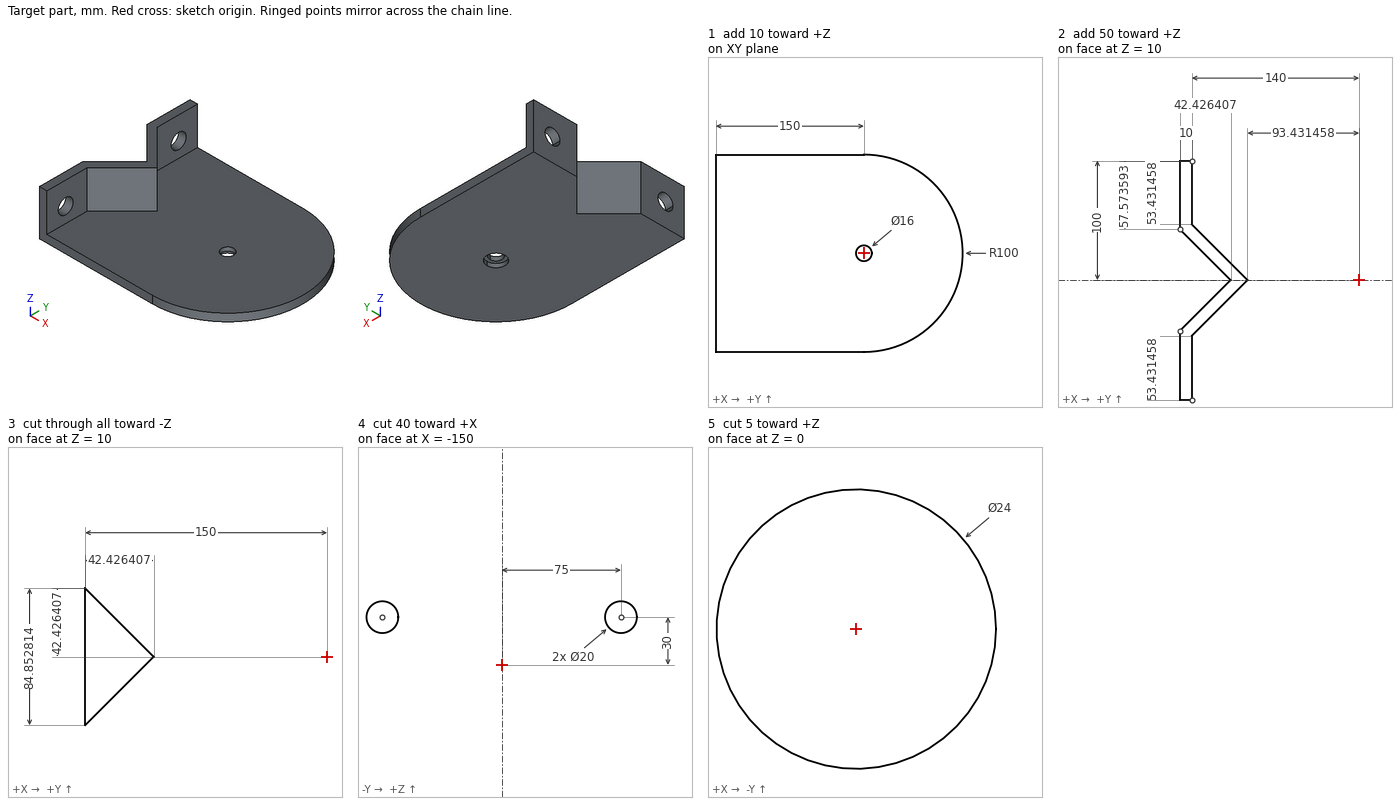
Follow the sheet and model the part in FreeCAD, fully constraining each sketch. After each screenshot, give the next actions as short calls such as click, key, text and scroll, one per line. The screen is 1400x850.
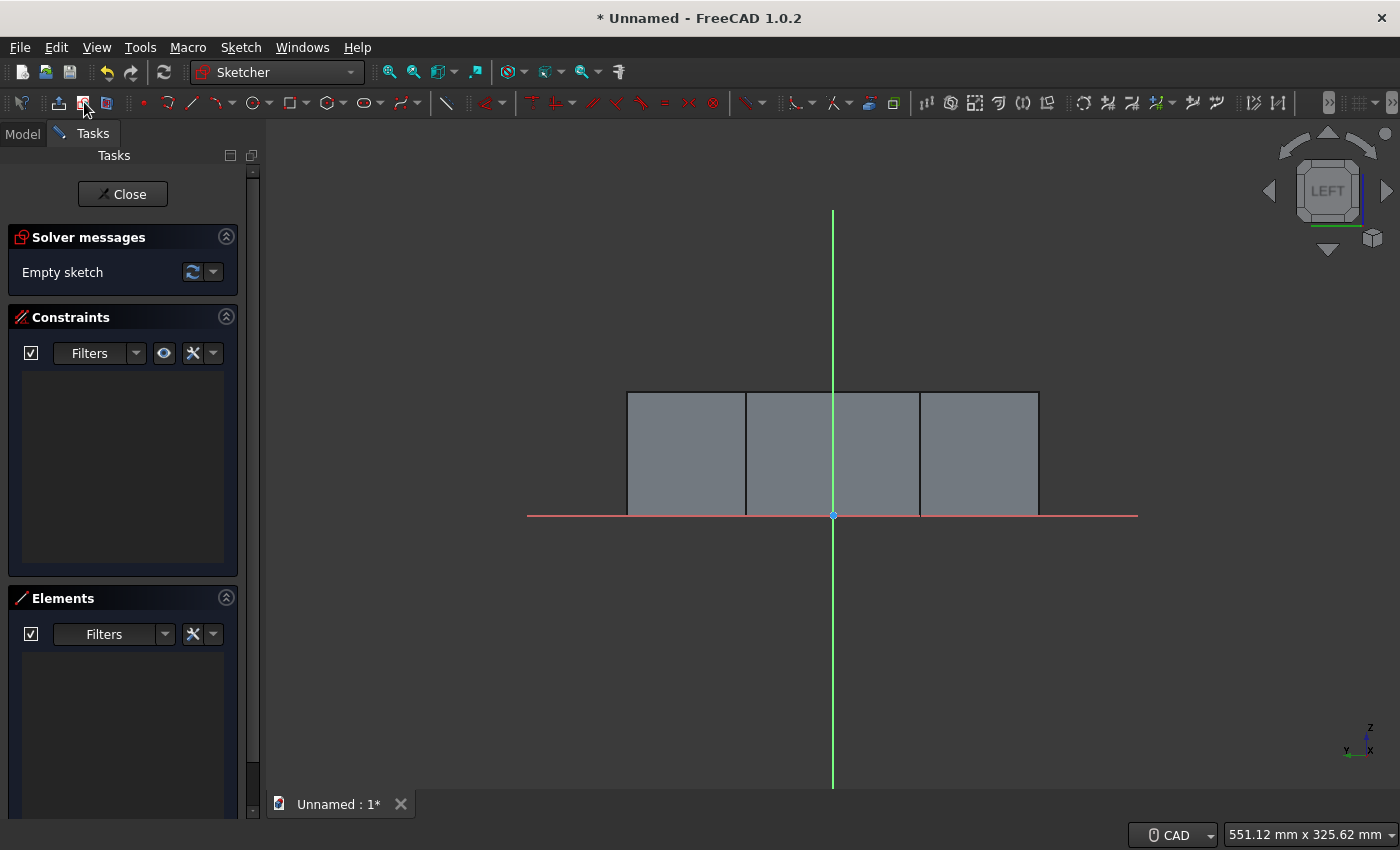
scroll(916, 500, up, 3)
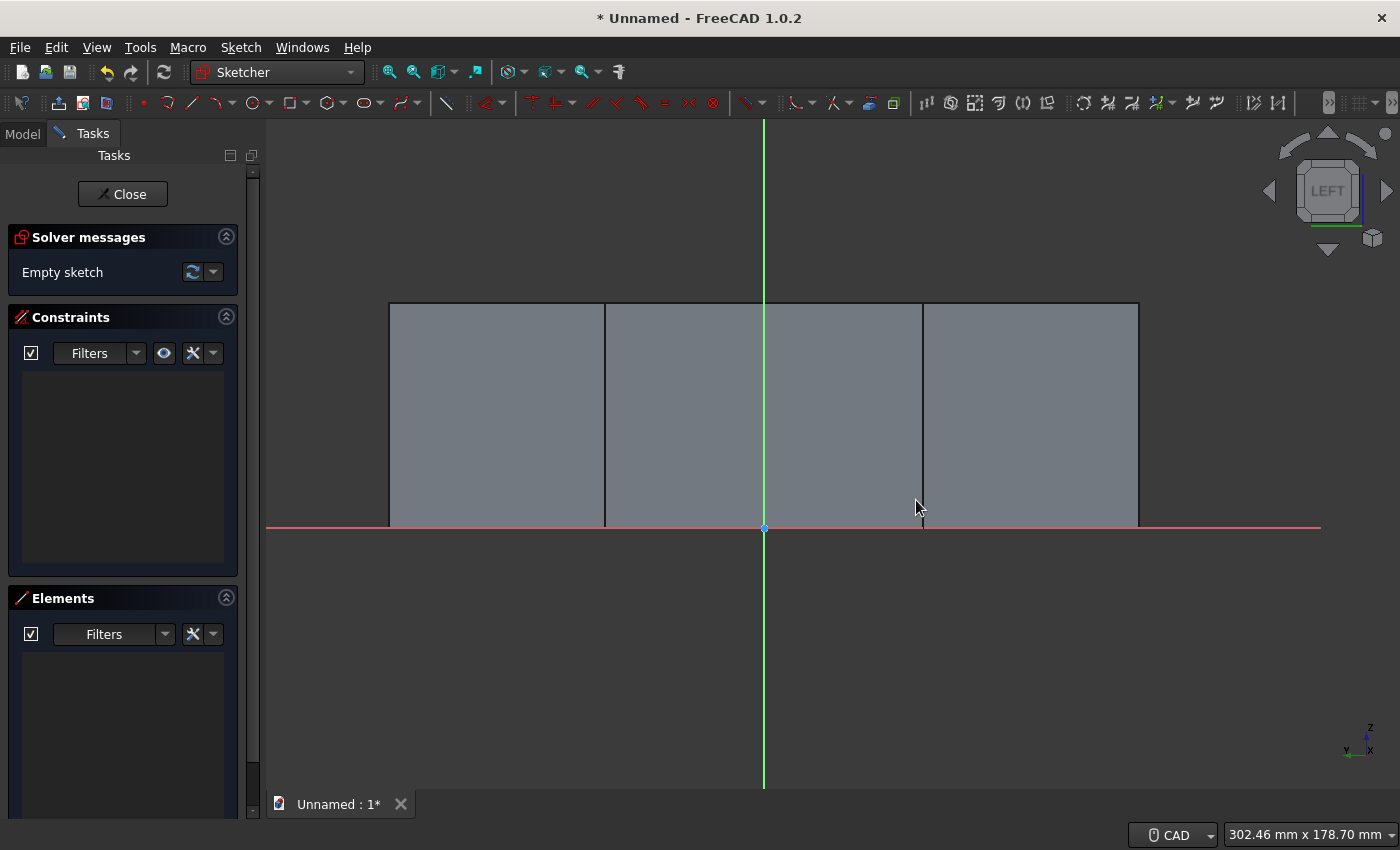
click(254, 104)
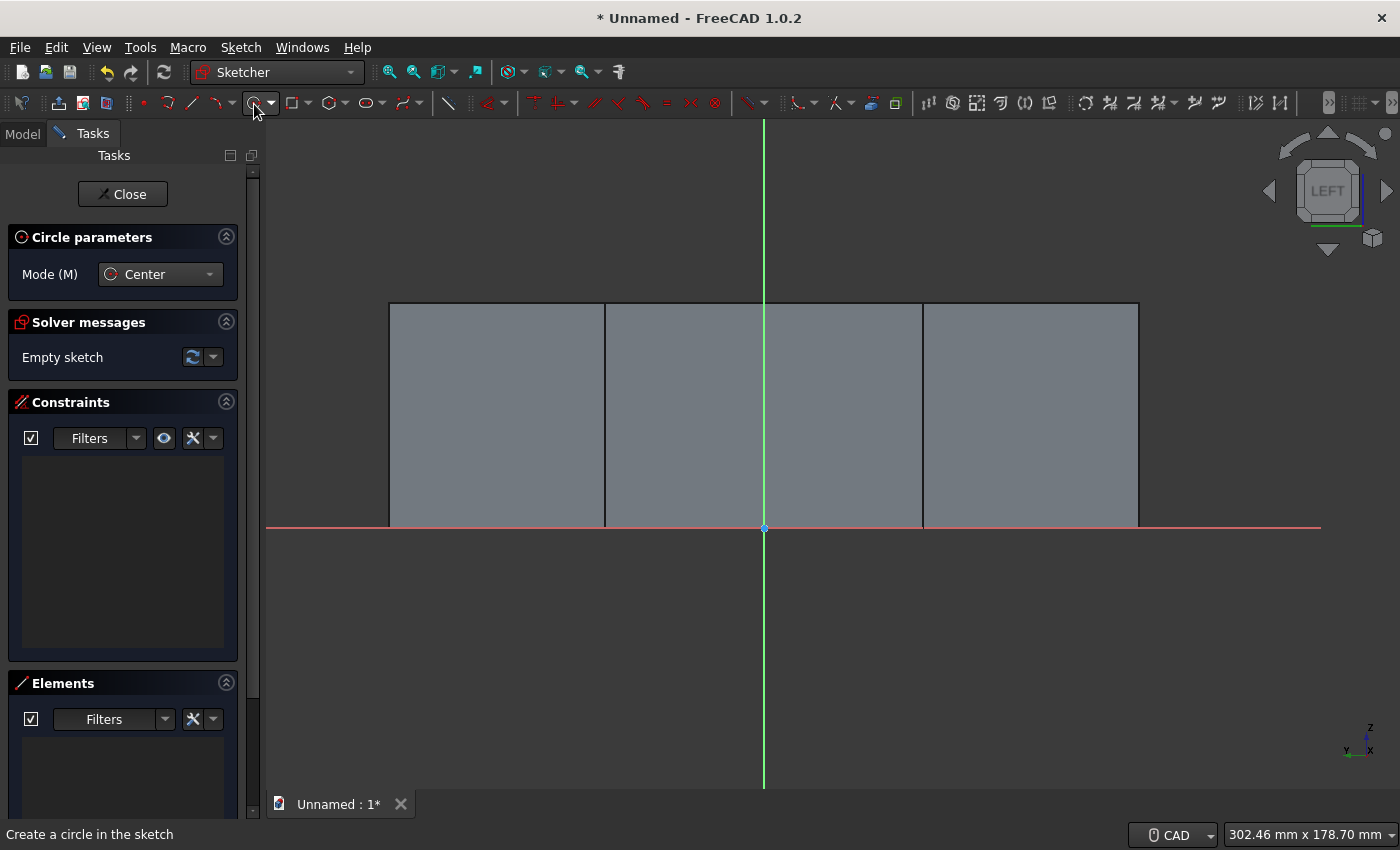
click(1045, 416)
click(1072, 389)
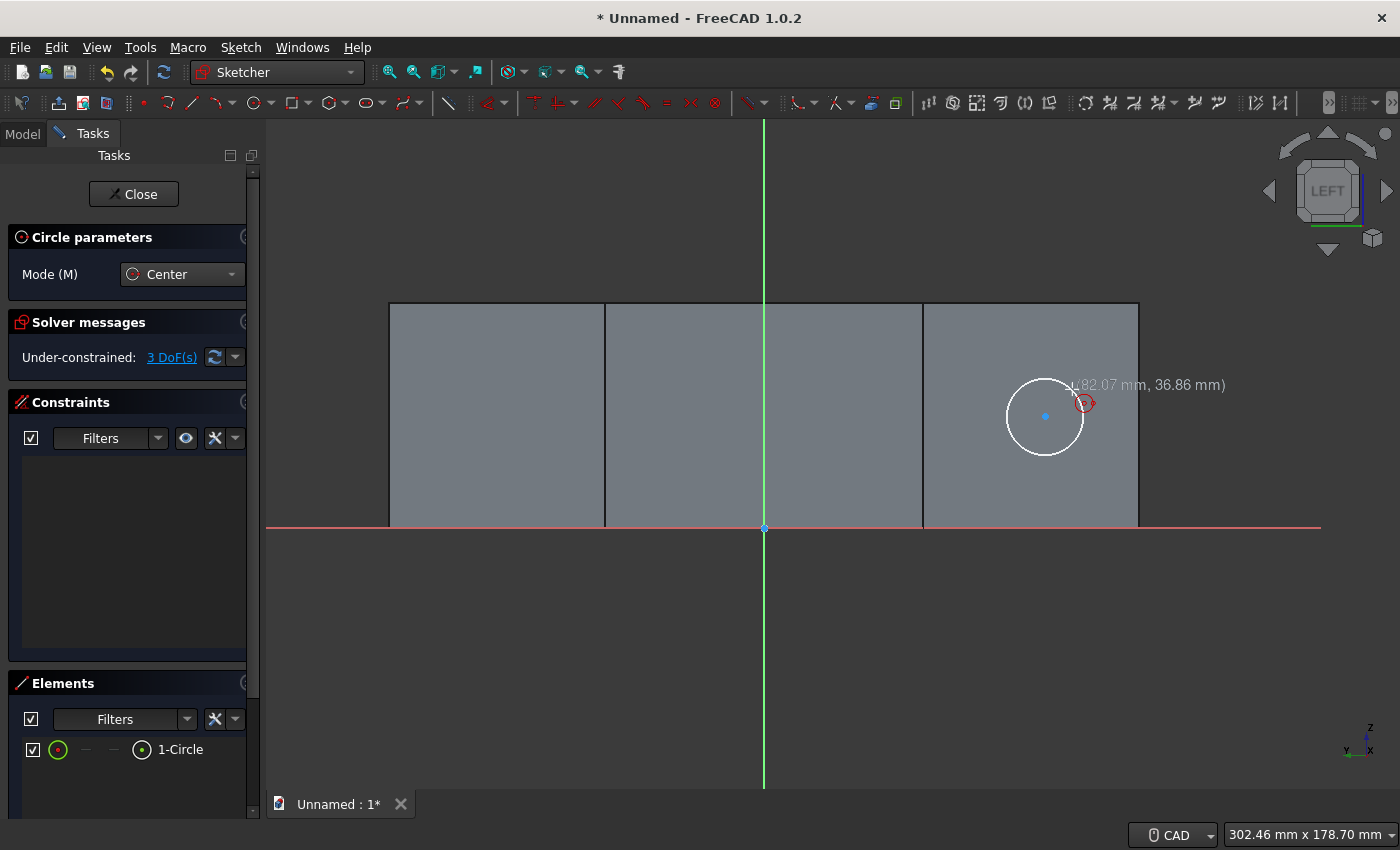
click(483, 416)
click(510, 389)
key(Escape)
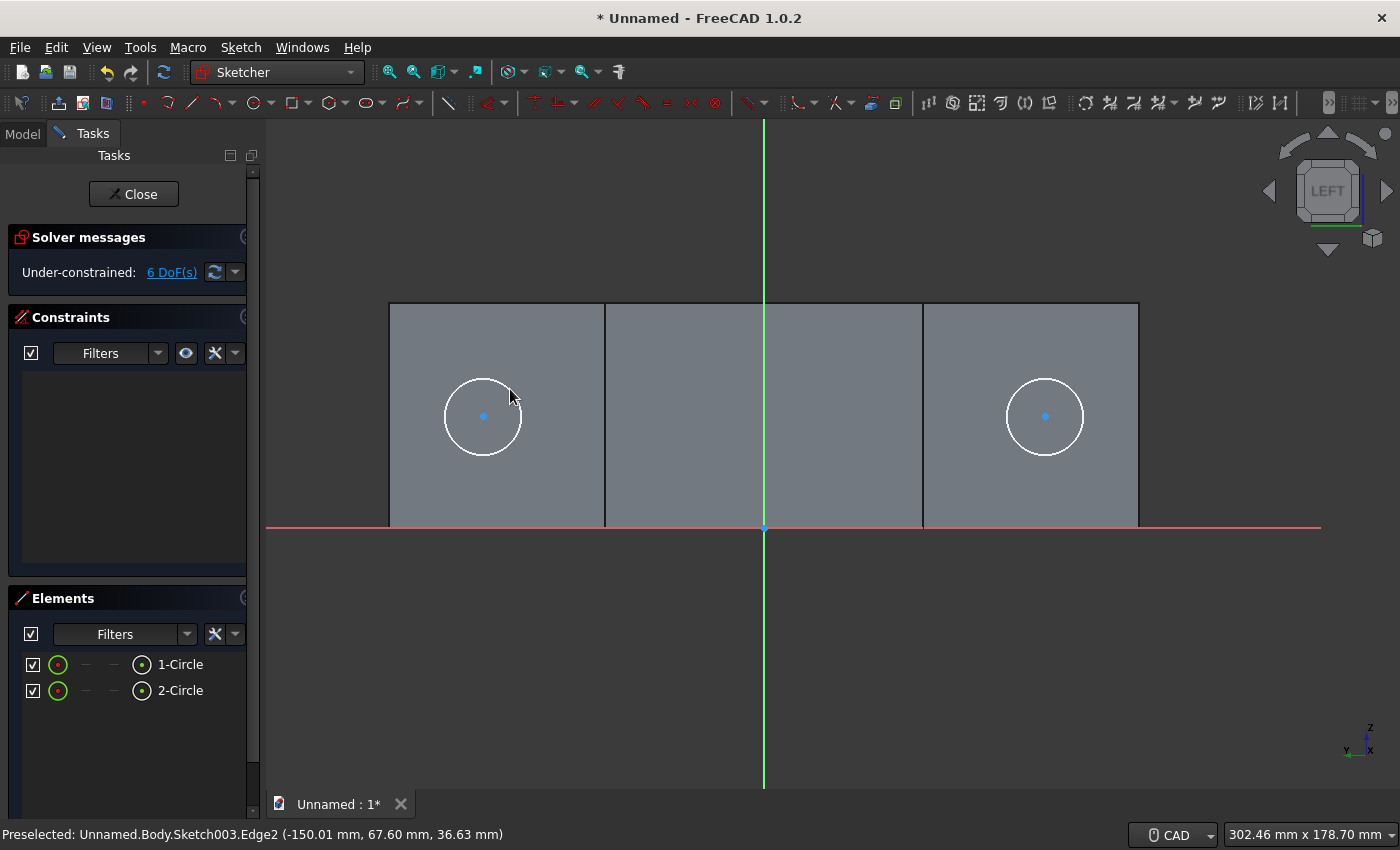
click(1072, 390)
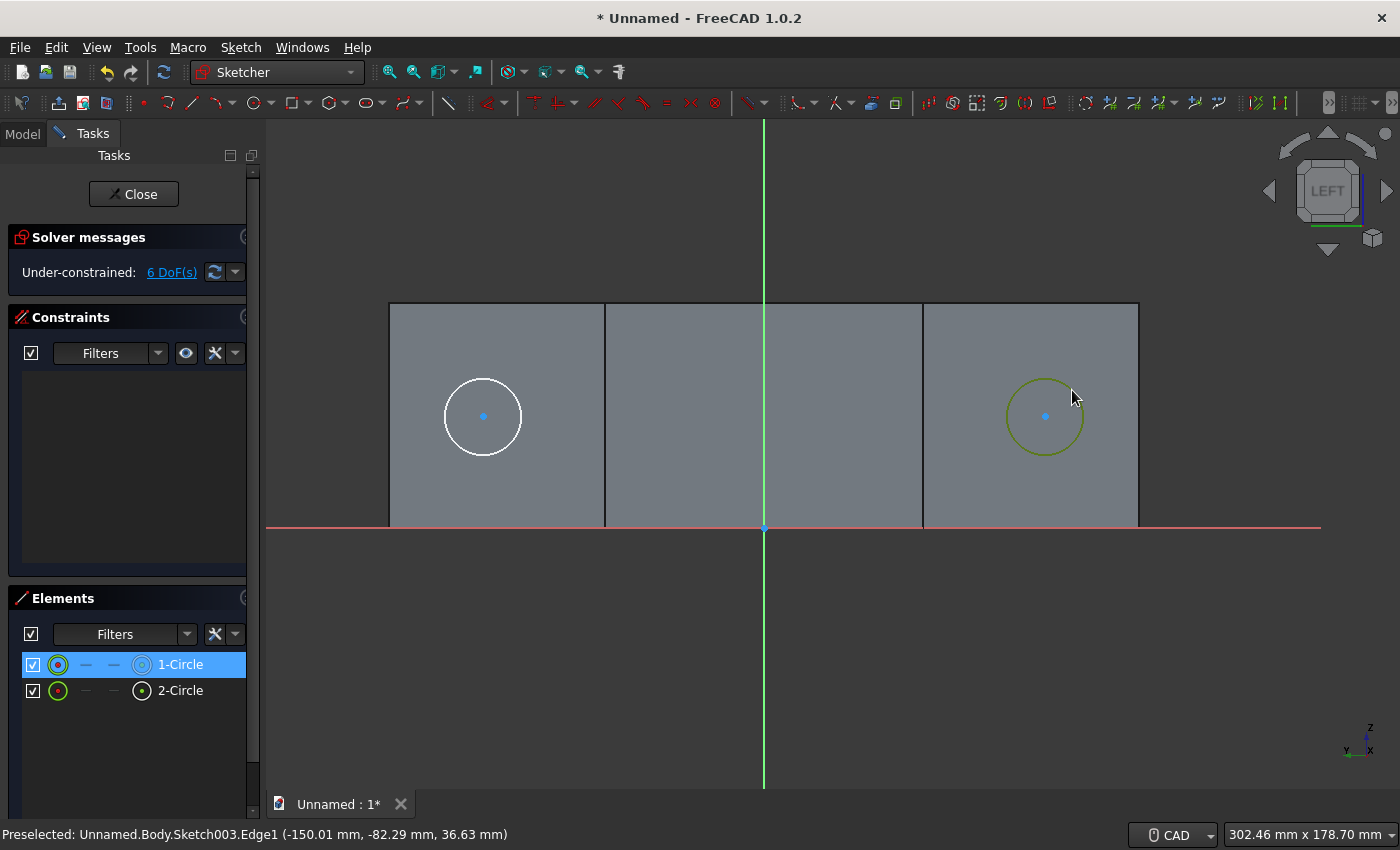
click(510, 390)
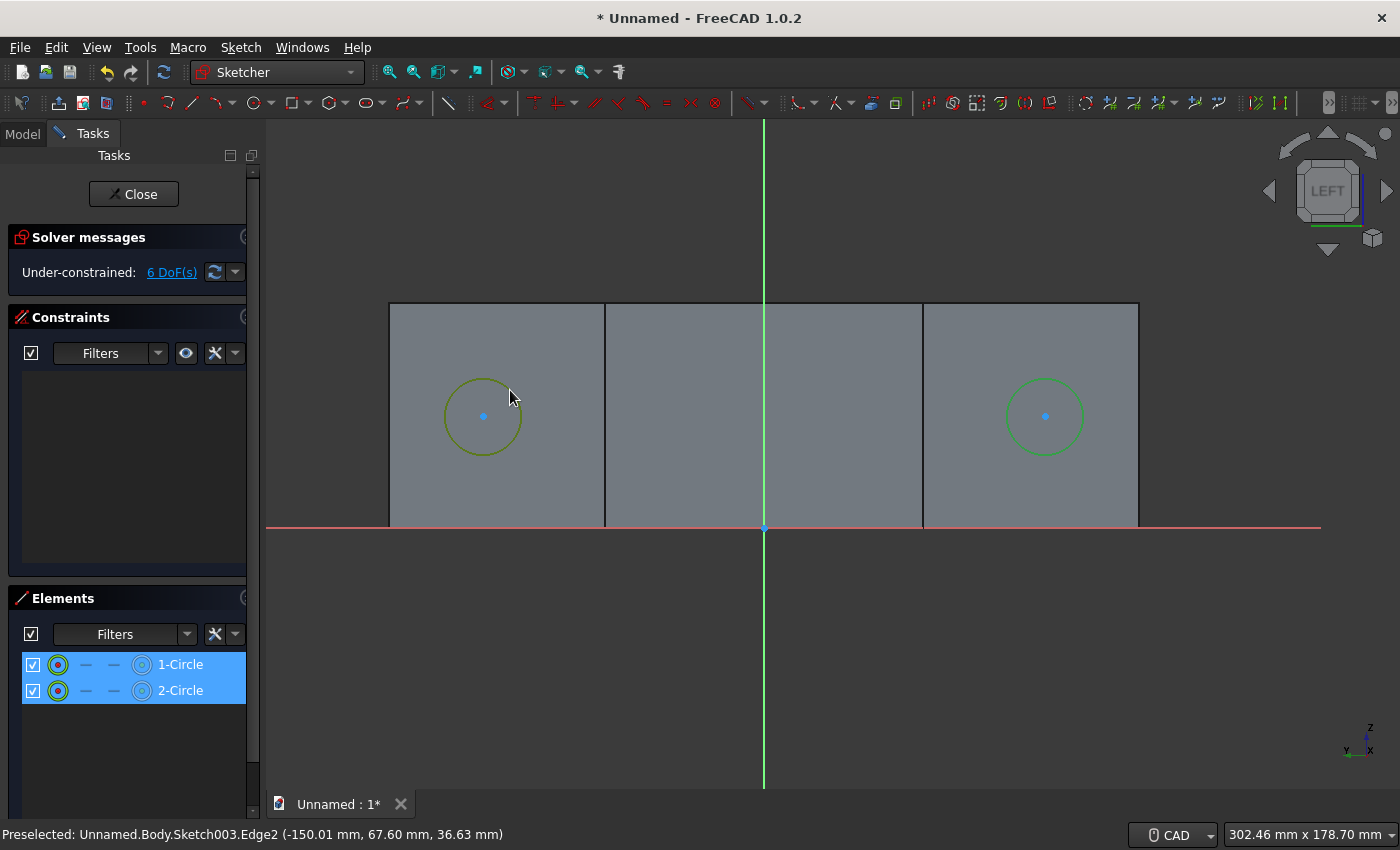
click(668, 104)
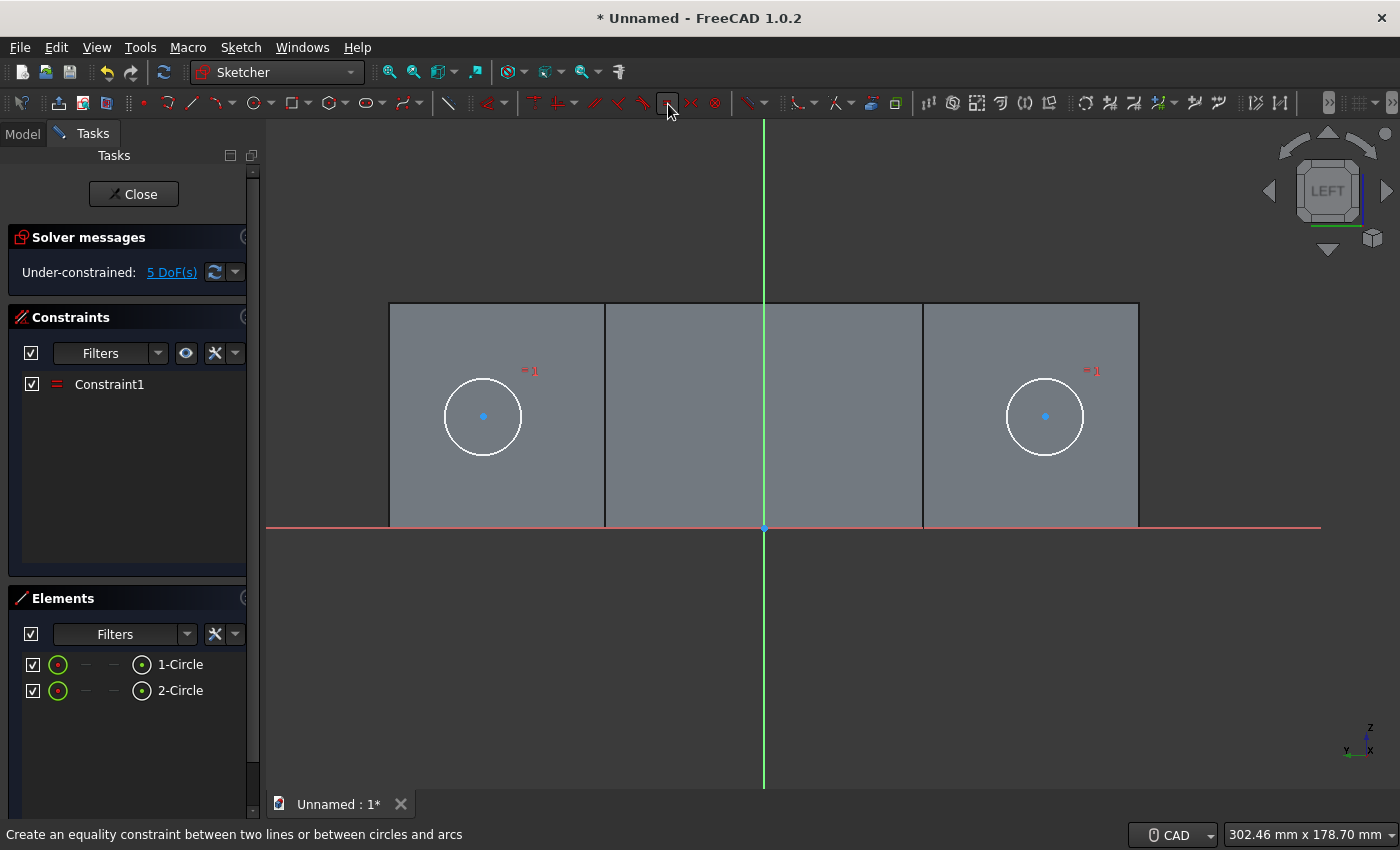
click(1045, 417)